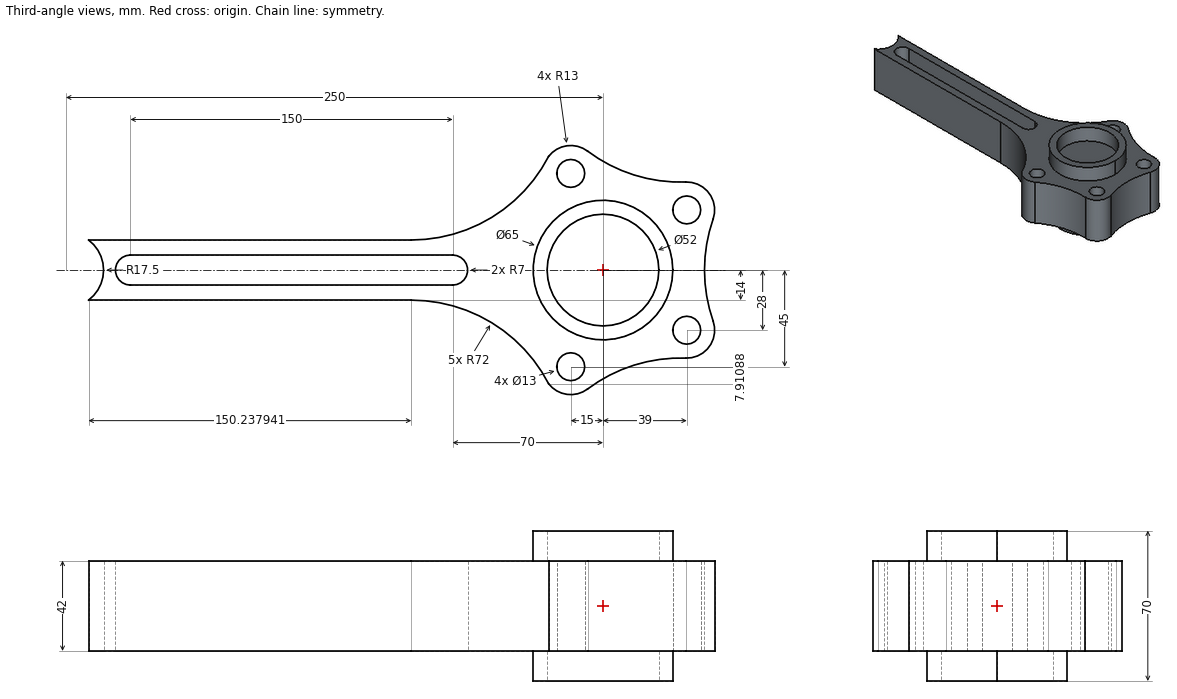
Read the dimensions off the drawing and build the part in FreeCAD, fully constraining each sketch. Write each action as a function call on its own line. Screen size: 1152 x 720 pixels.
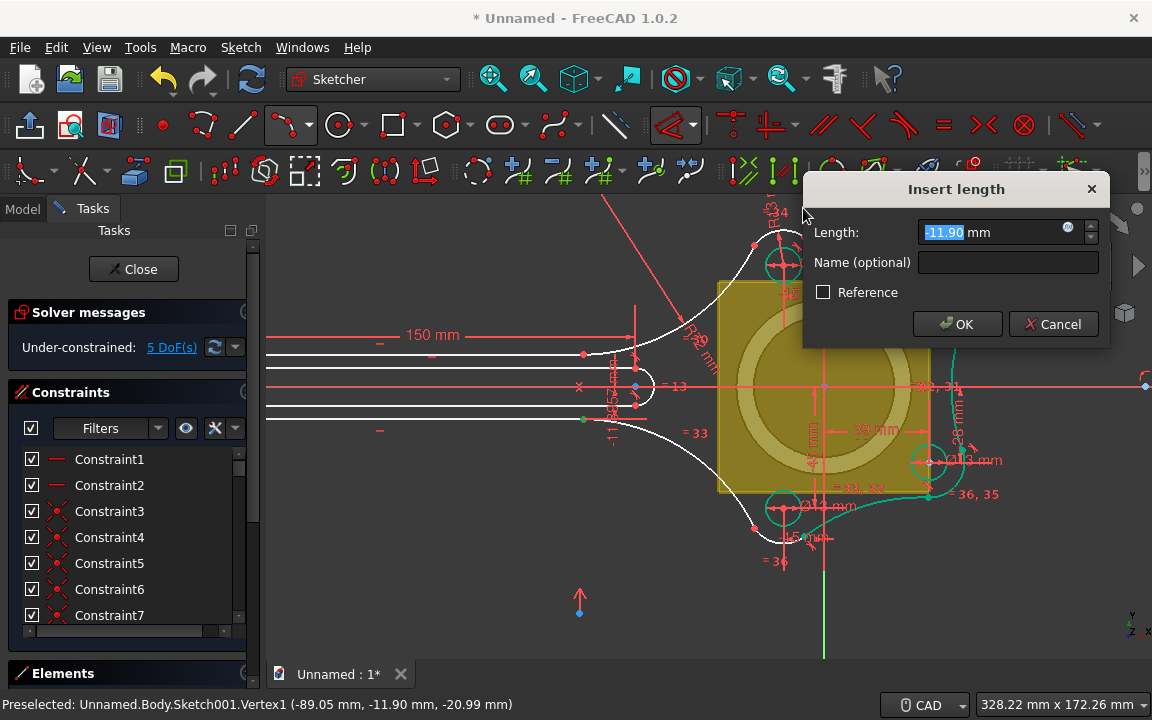
text(-14)
key(Return)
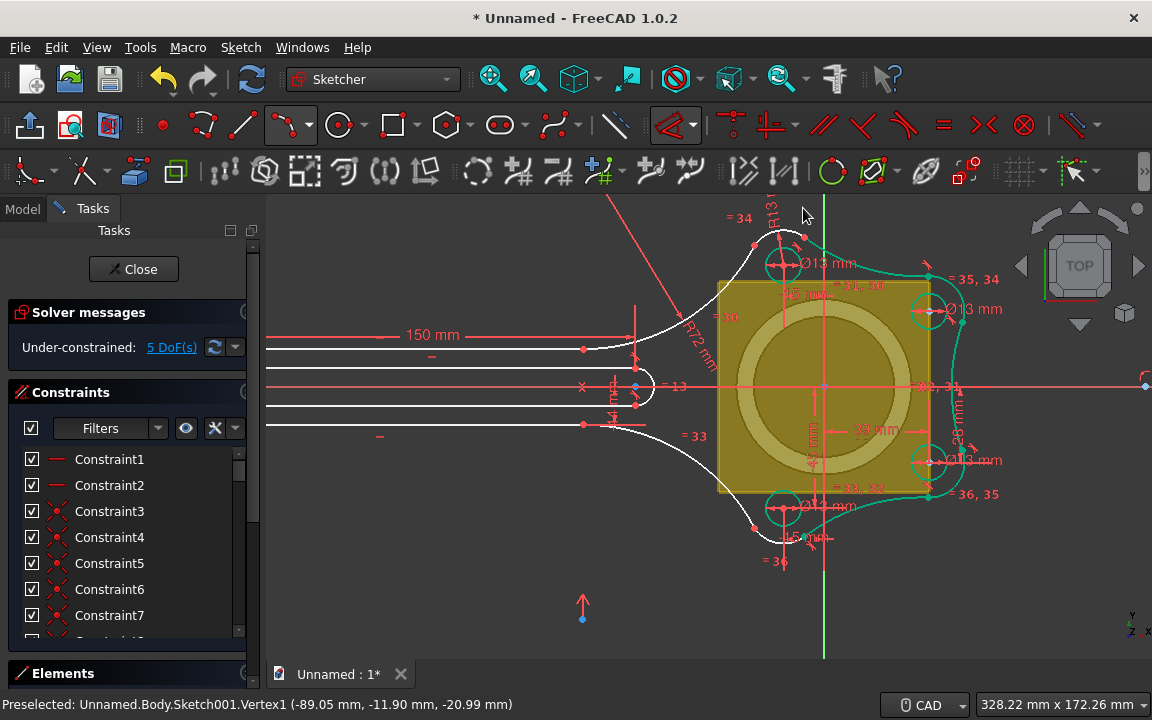
click(635, 406)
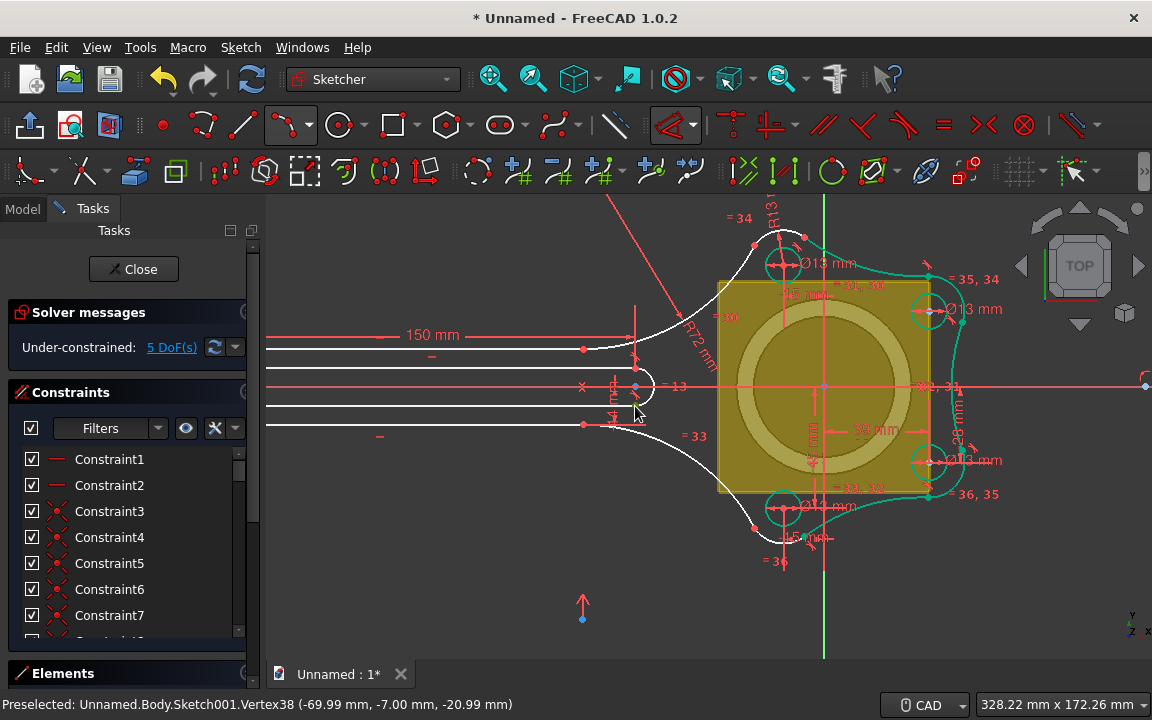
click(696, 126)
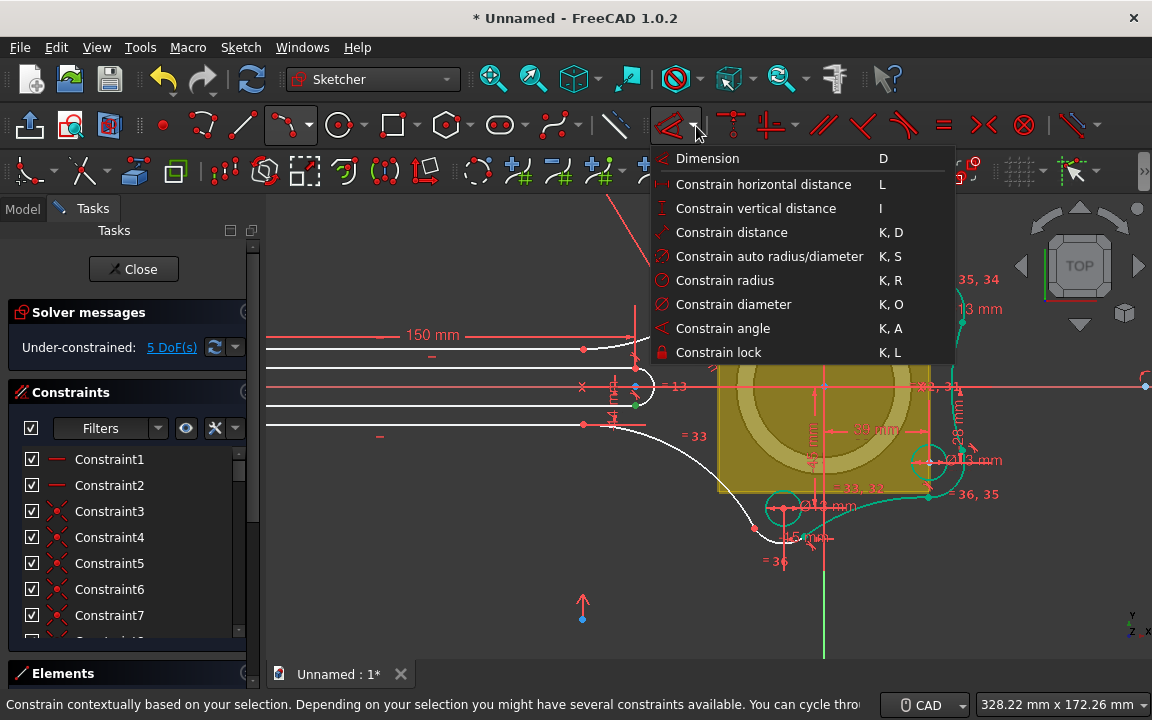
click(803, 184)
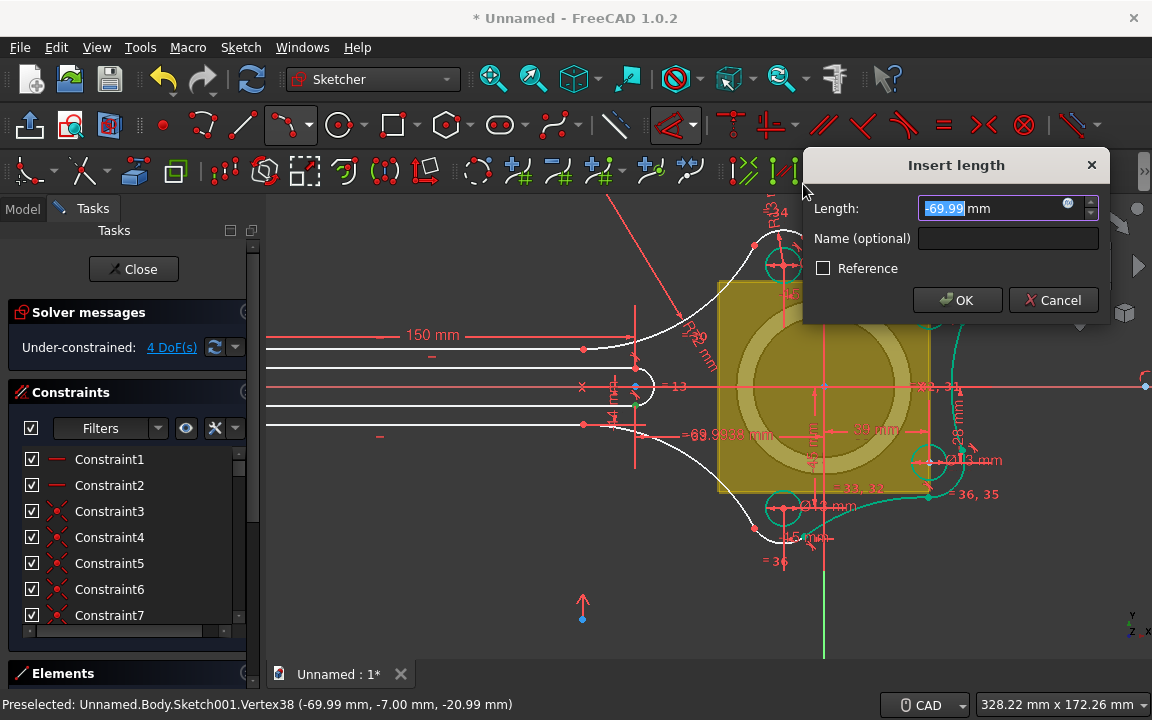
text(-70)
key(Return)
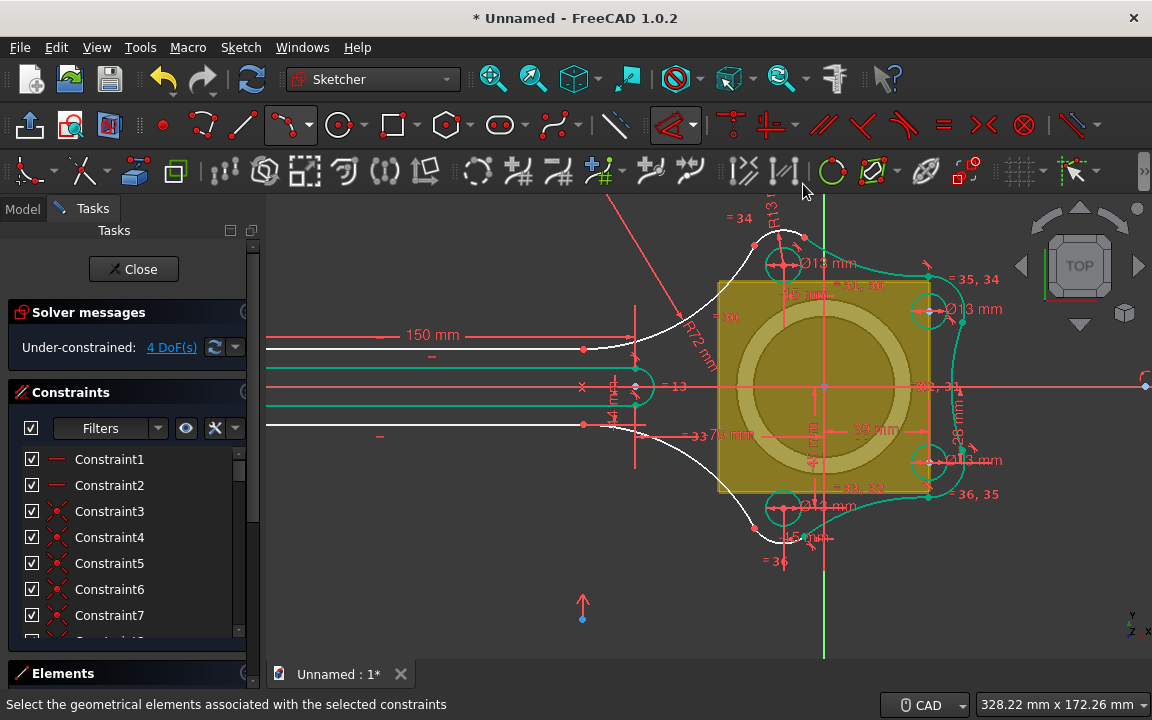
scroll(784, 507, down, 2)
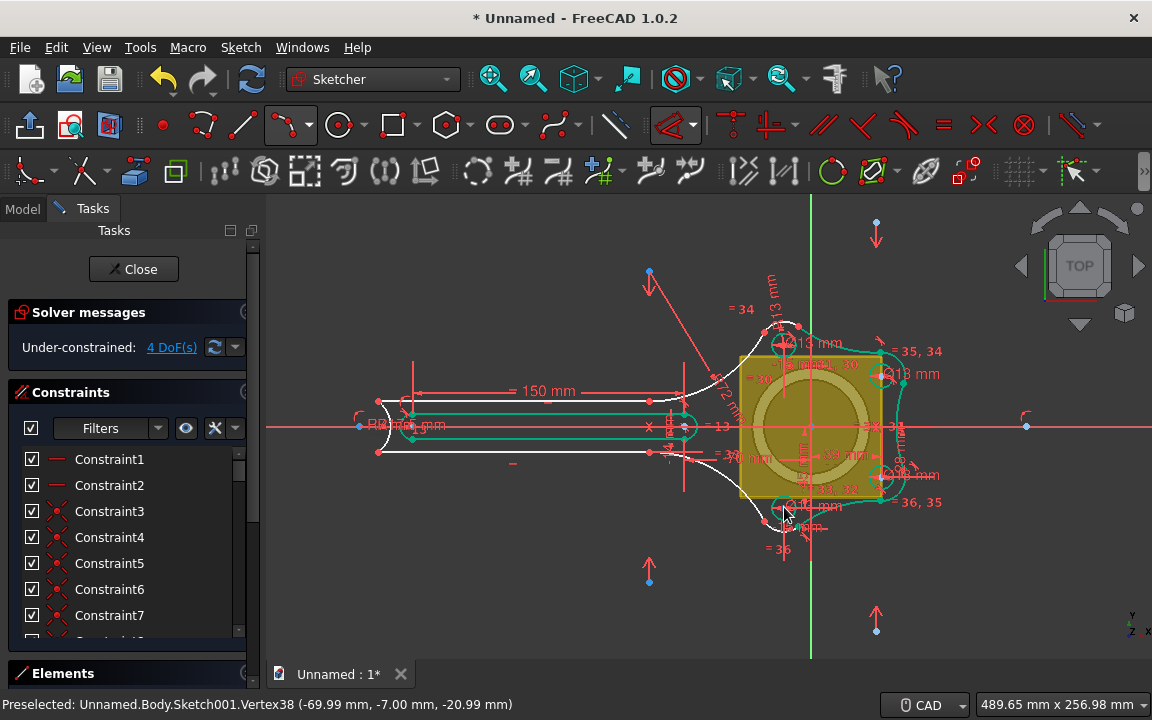
click(359, 427)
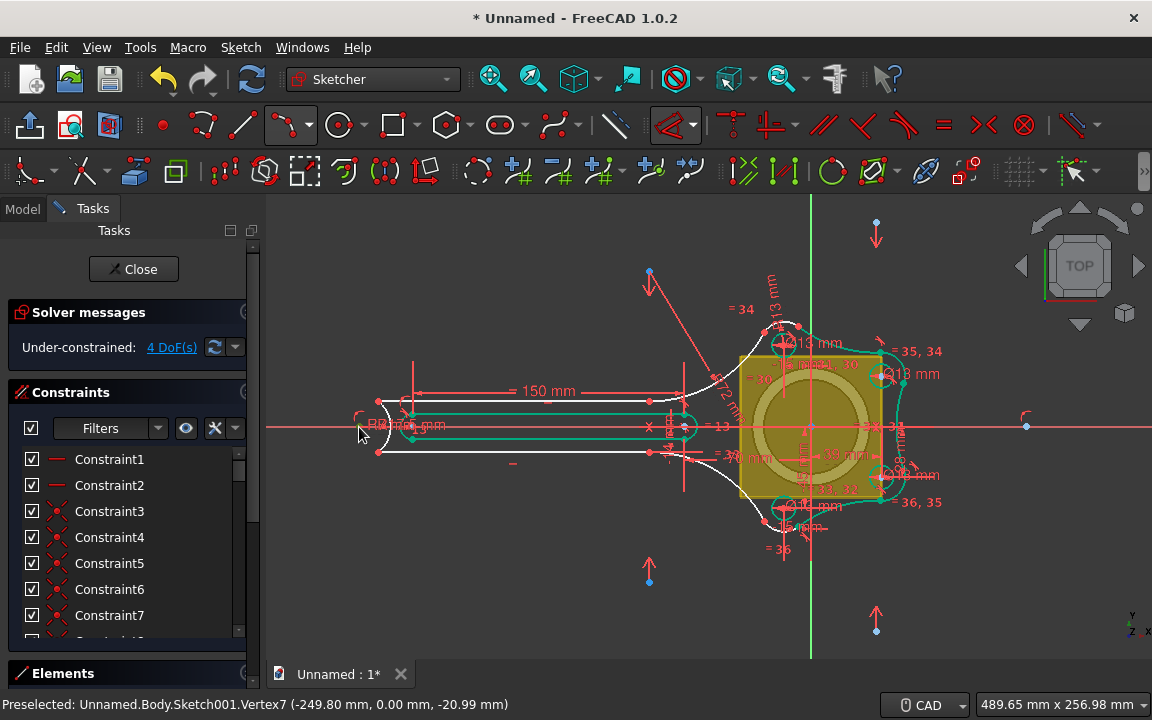
click(696, 126)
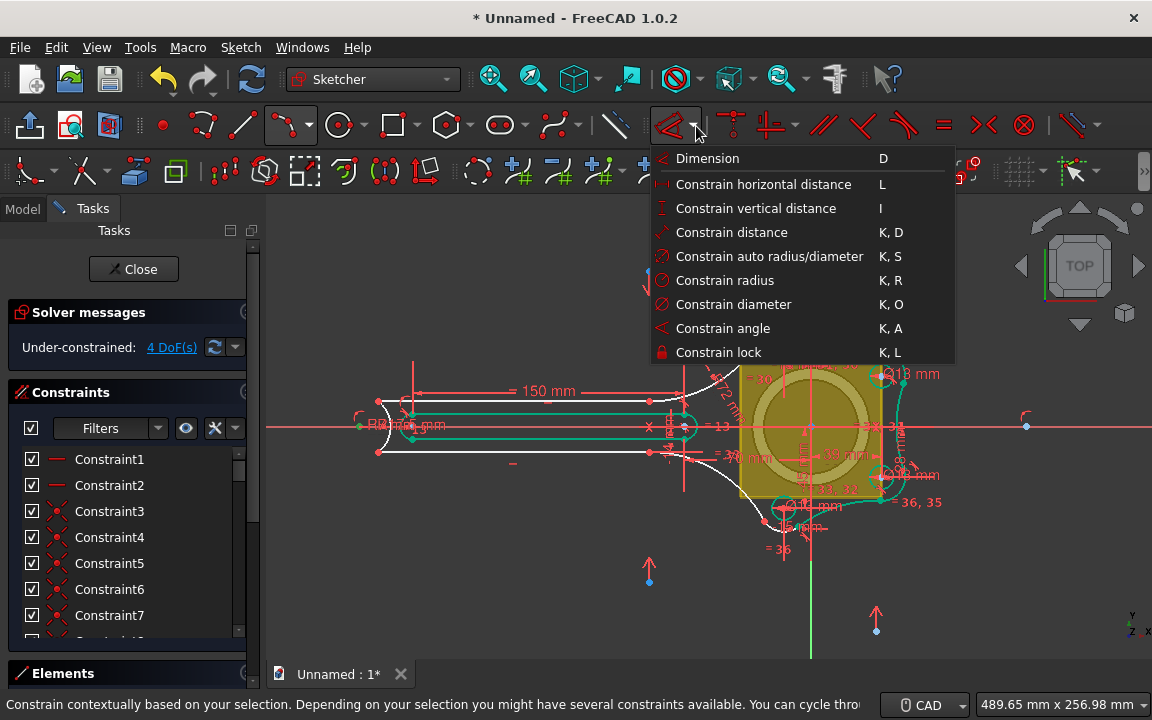
click(803, 184)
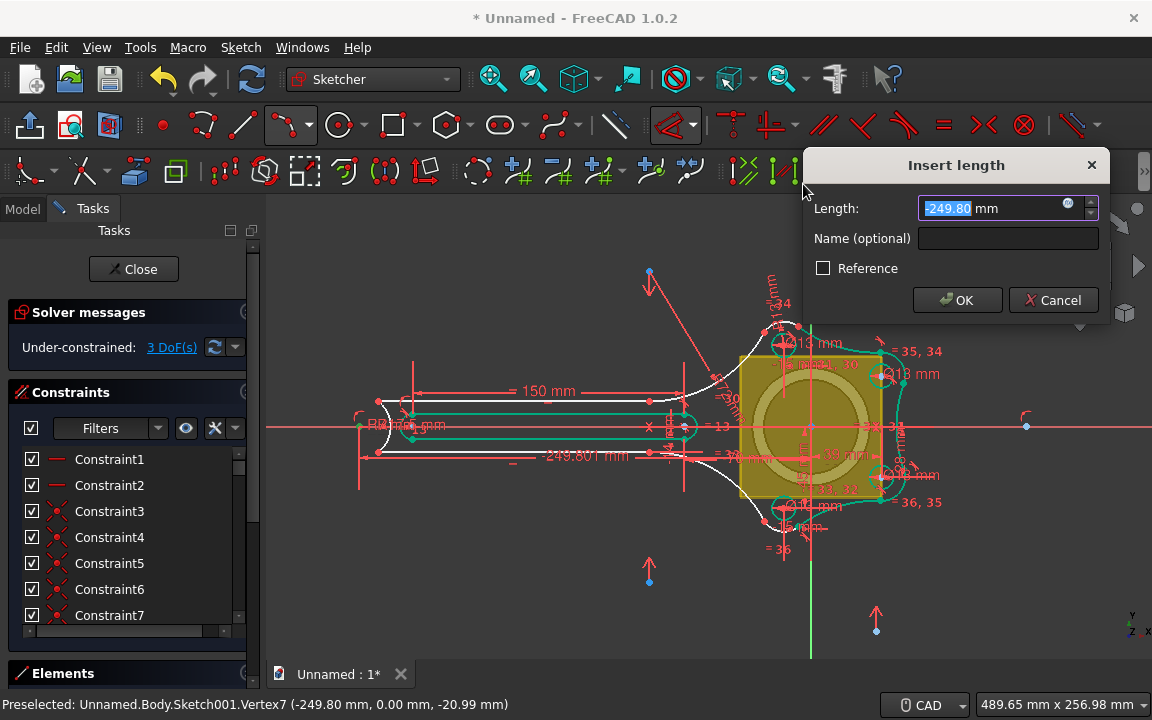
text(-250)
key(Return)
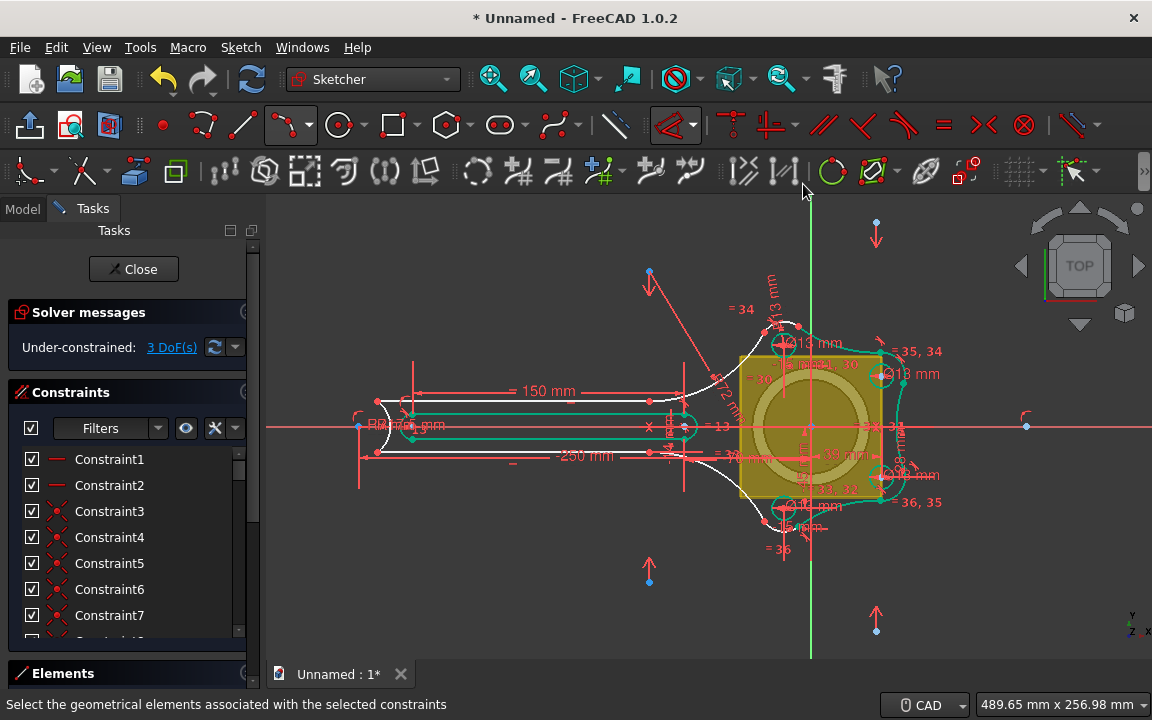
scroll(764, 521, up, 6)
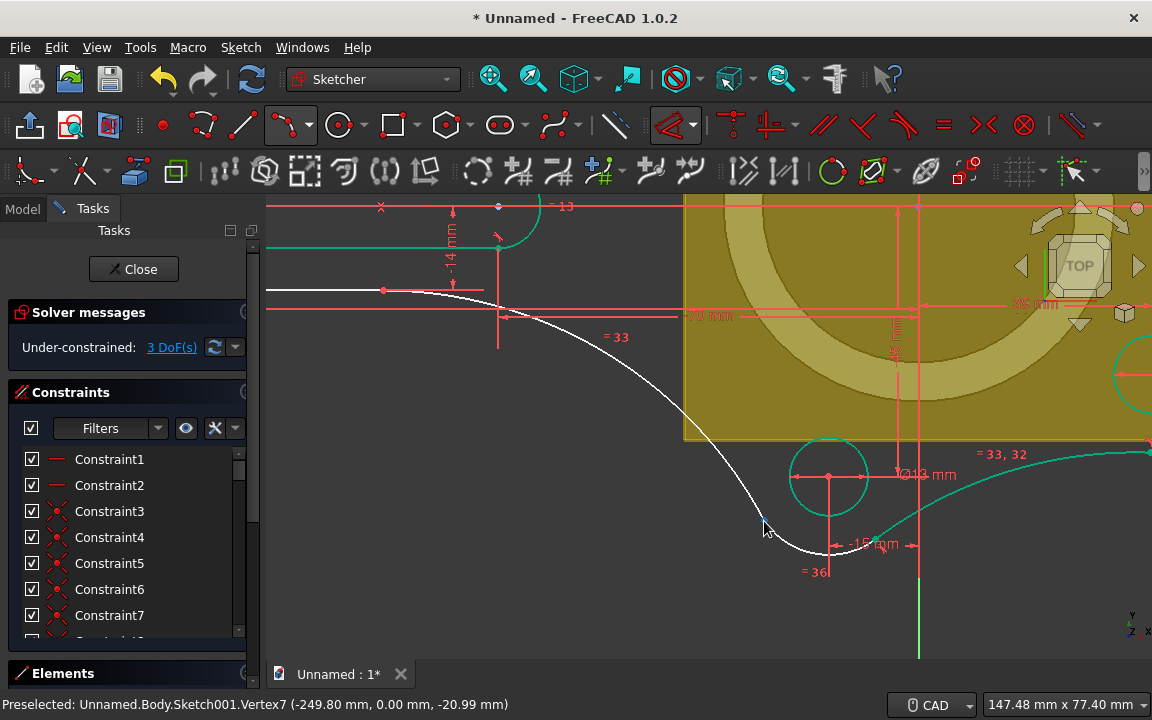
click(764, 521)